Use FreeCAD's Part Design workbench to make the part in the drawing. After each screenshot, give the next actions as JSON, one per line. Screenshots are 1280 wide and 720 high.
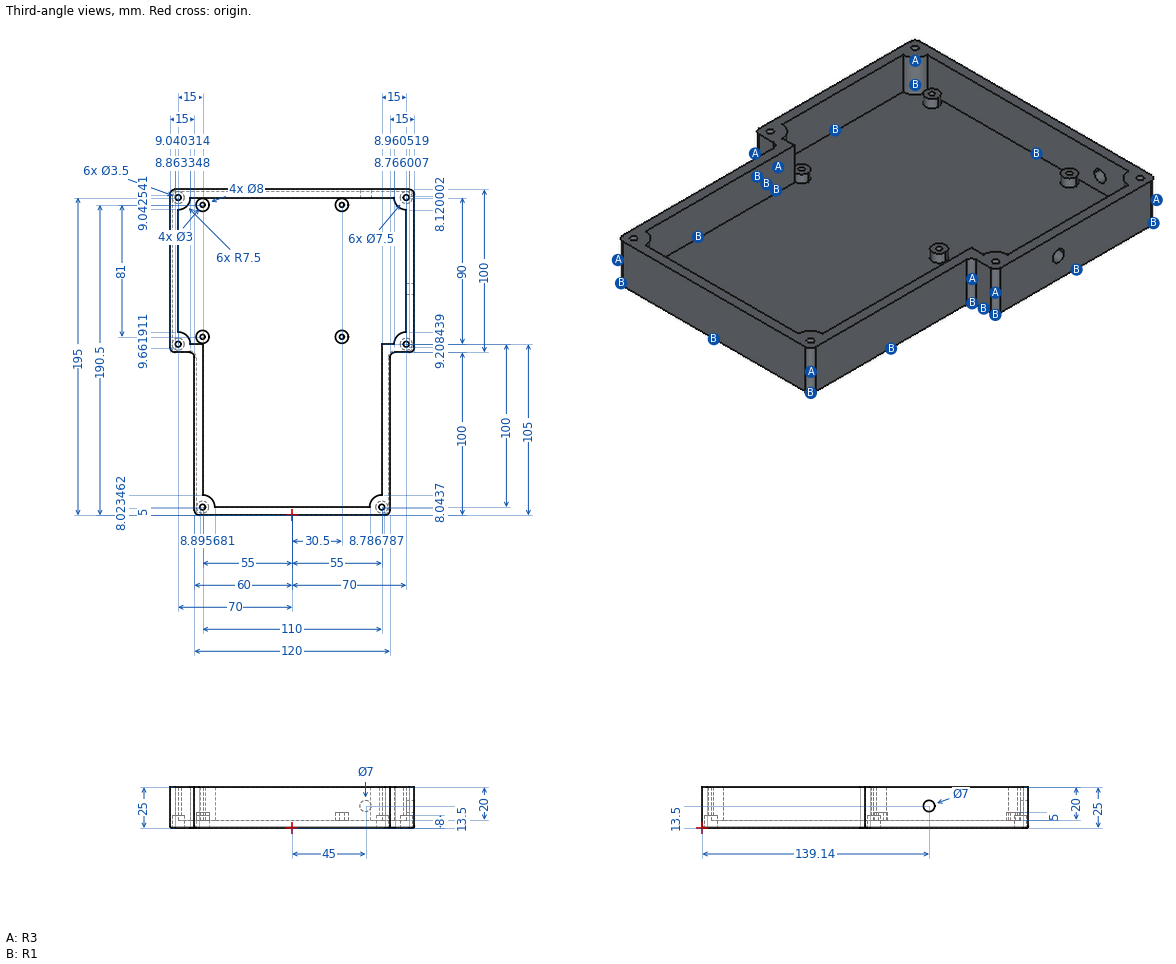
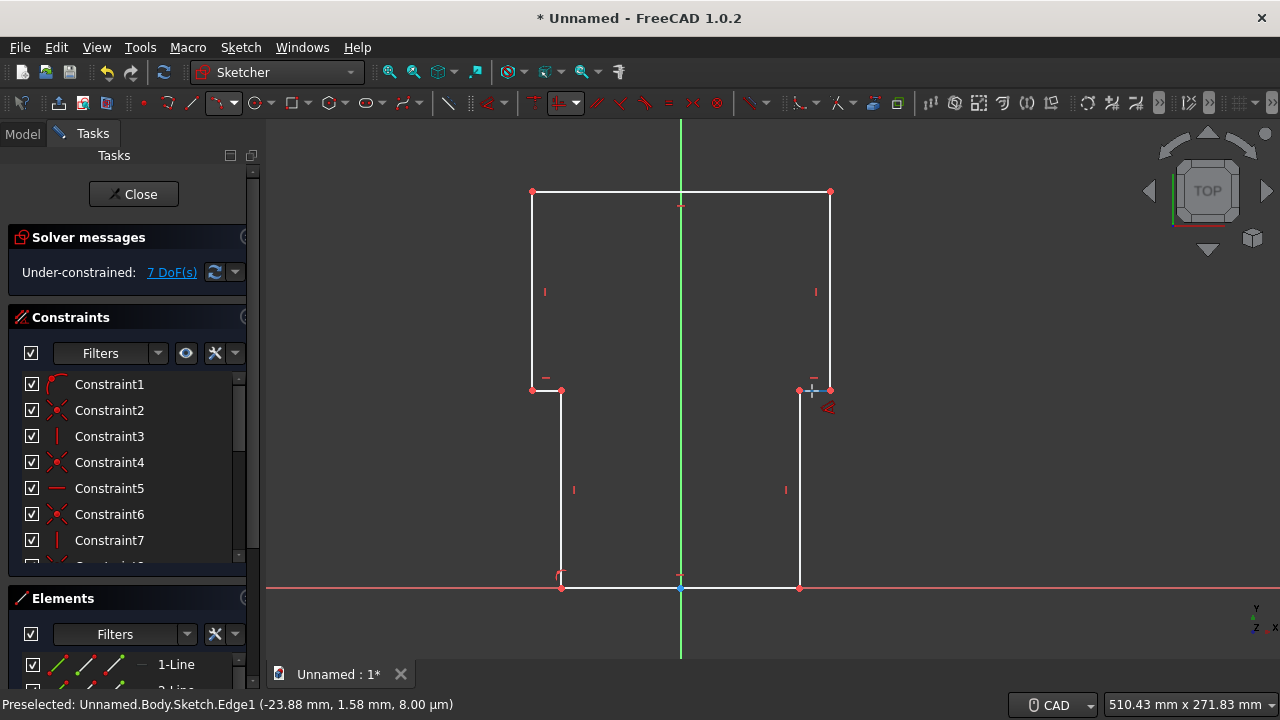
{"action": "left_click", "coordinate": [812, 391]}
{"action": "left_click", "coordinate": [816, 425]}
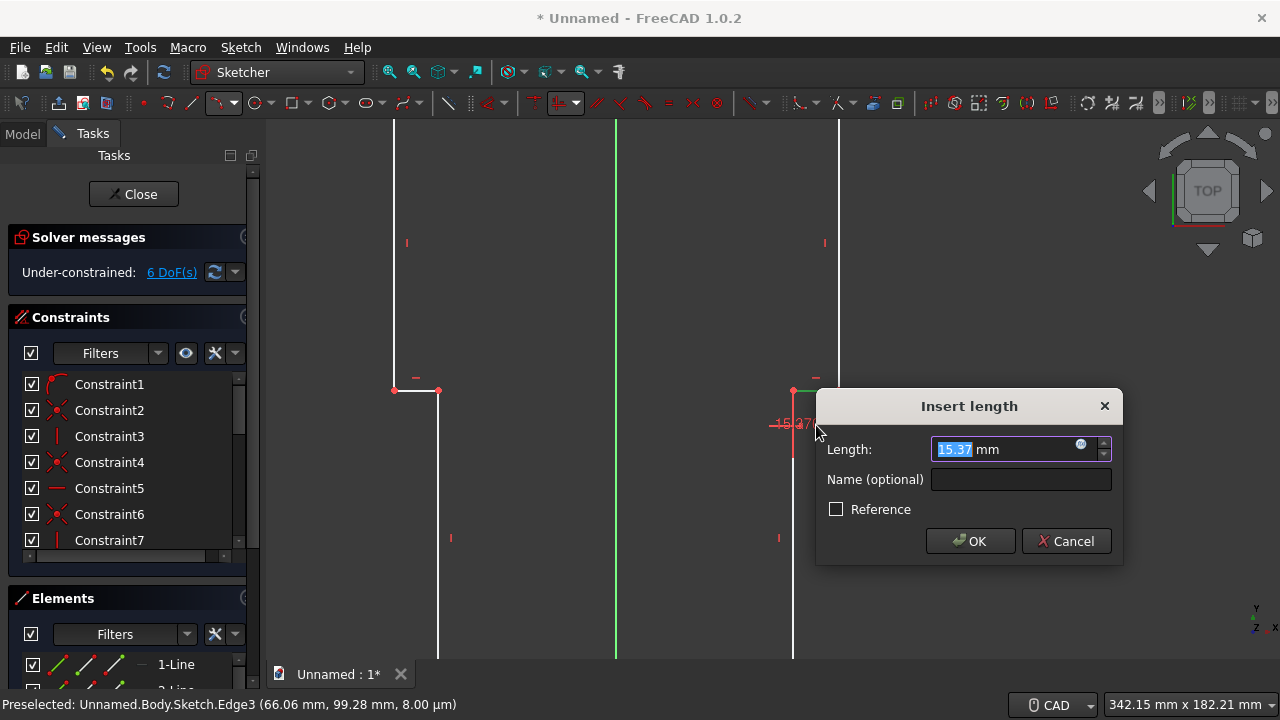
{"action": "type", "text": "15"}
{"action": "key", "text": "Return"}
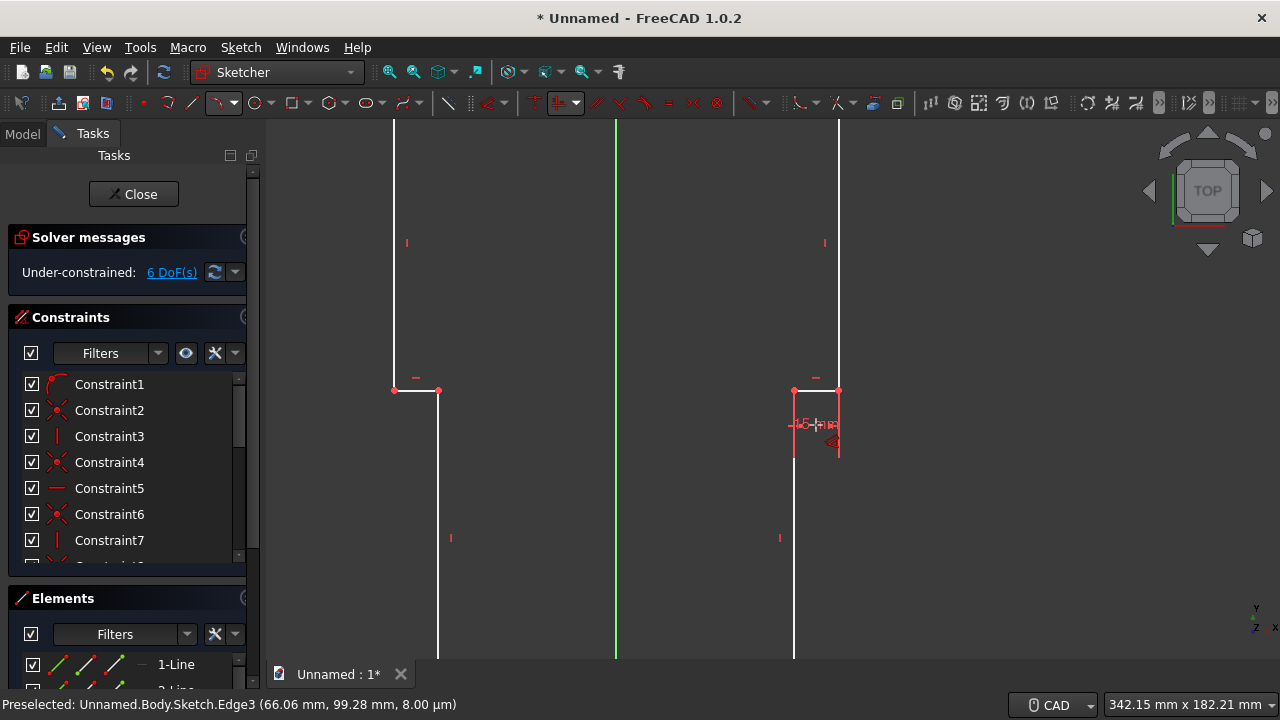
{"action": "left_click", "coordinate": [407, 391]}
{"action": "left_click", "coordinate": [416, 425]}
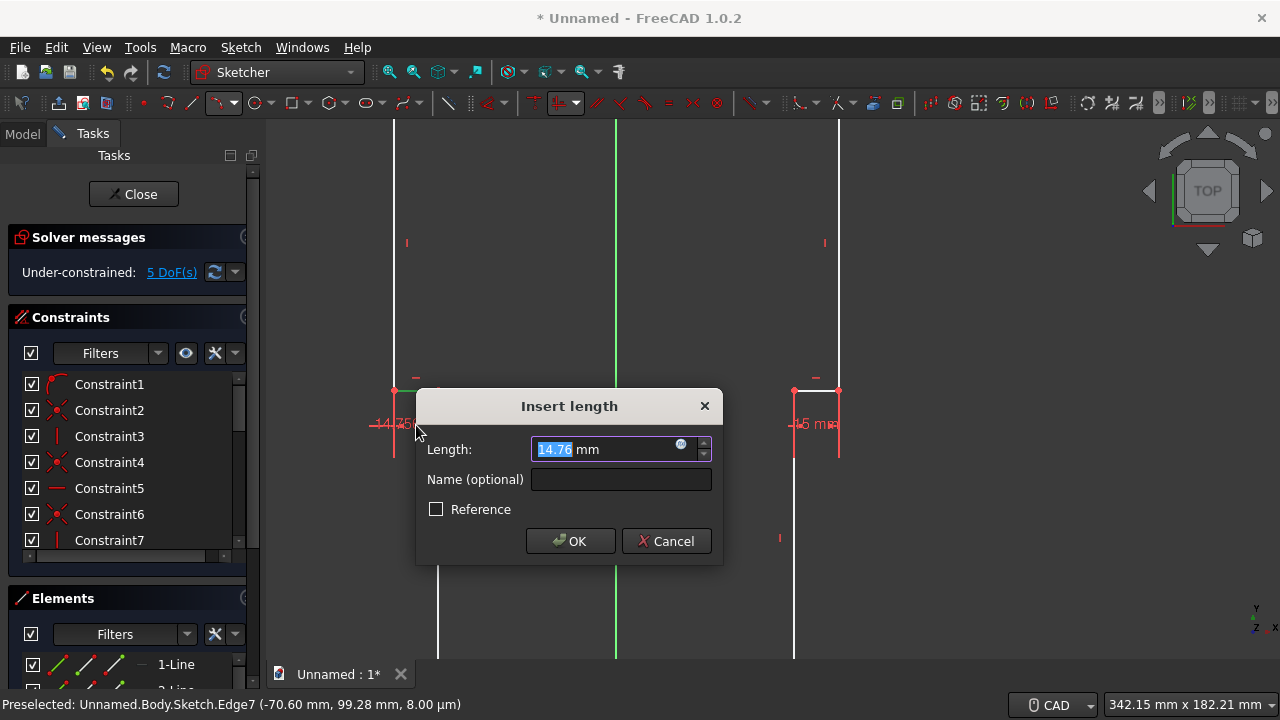
{"action": "type", "text": "15"}
{"action": "key", "text": "Return"}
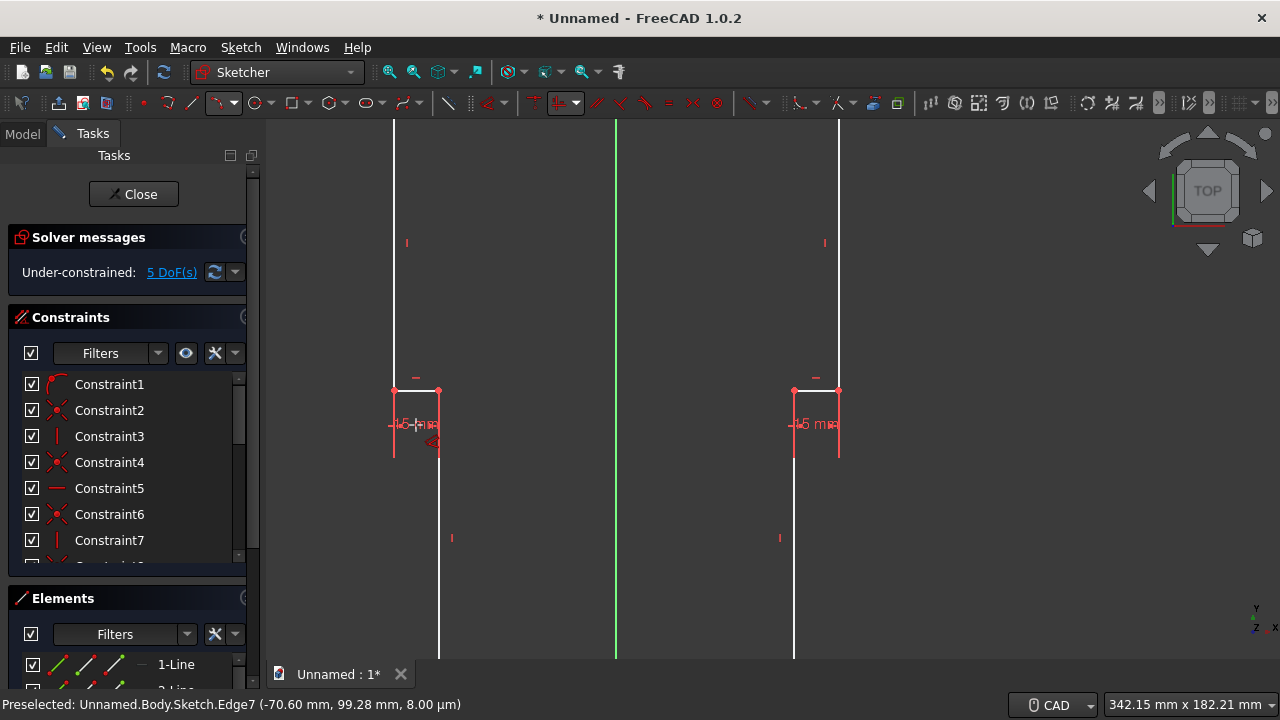
{"action": "scroll", "coordinate": [812, 390], "scroll_direction": "down", "scroll_amount": 3}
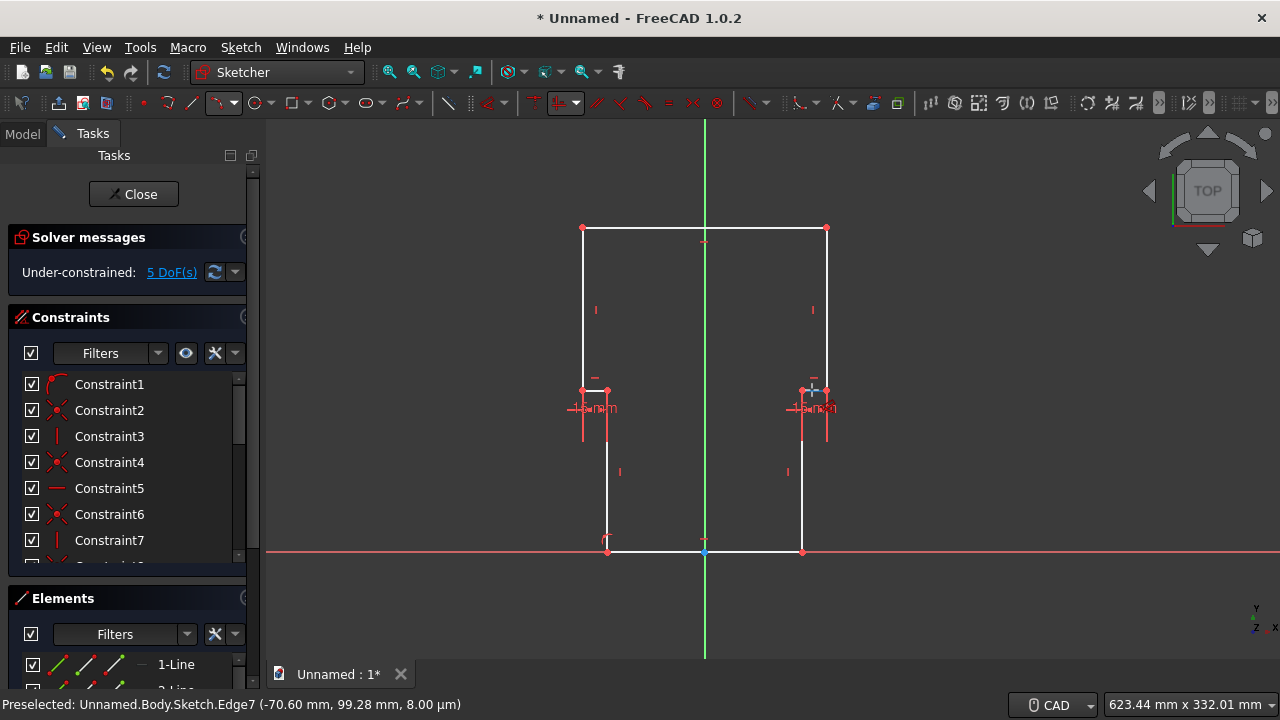
{"action": "left_click", "coordinate": [666, 552]}
{"action": "left_click", "coordinate": [660, 586]}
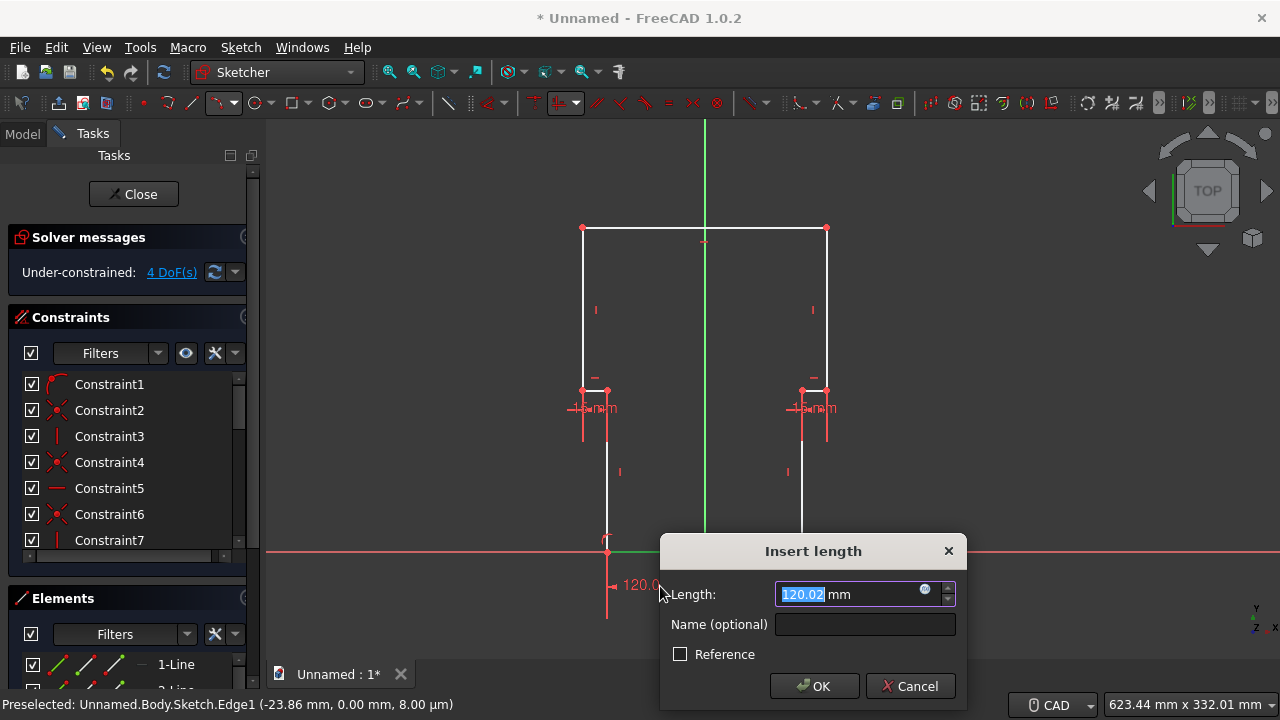
{"action": "type", "text": "120"}
{"action": "key", "text": "Return"}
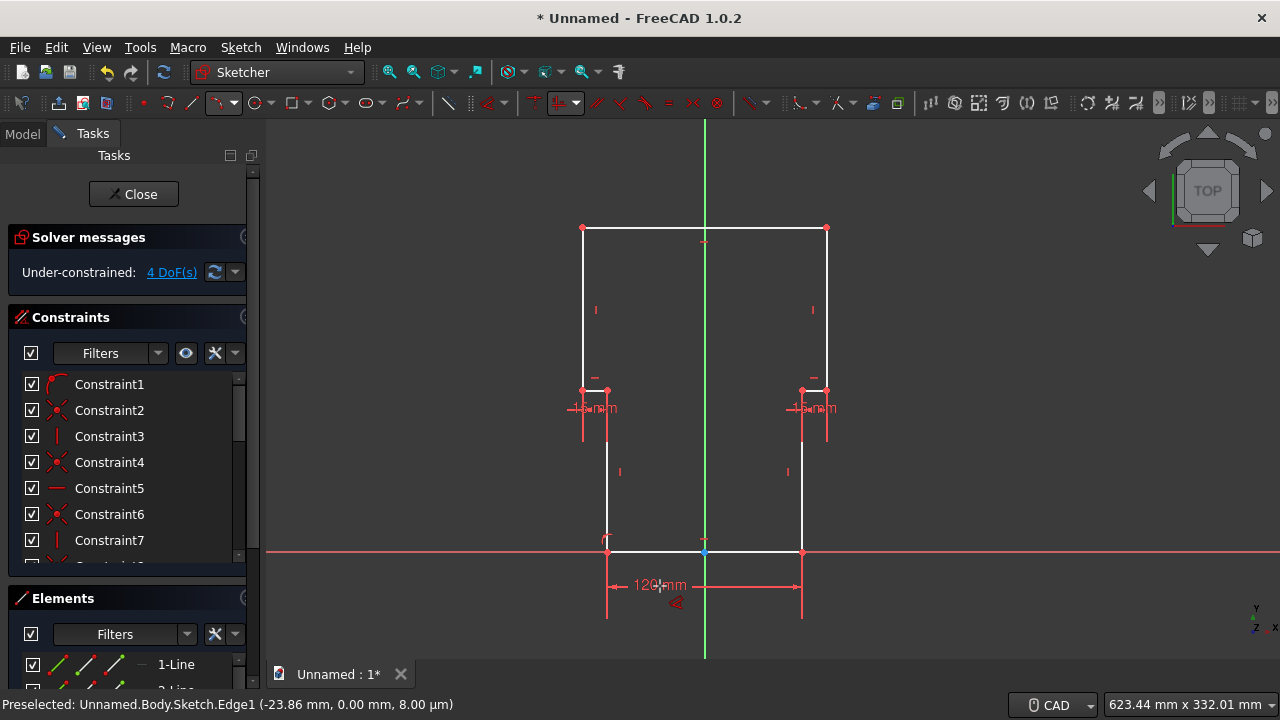
{"action": "left_click", "coordinate": [802, 504]}
{"action": "left_click", "coordinate": [836, 471]}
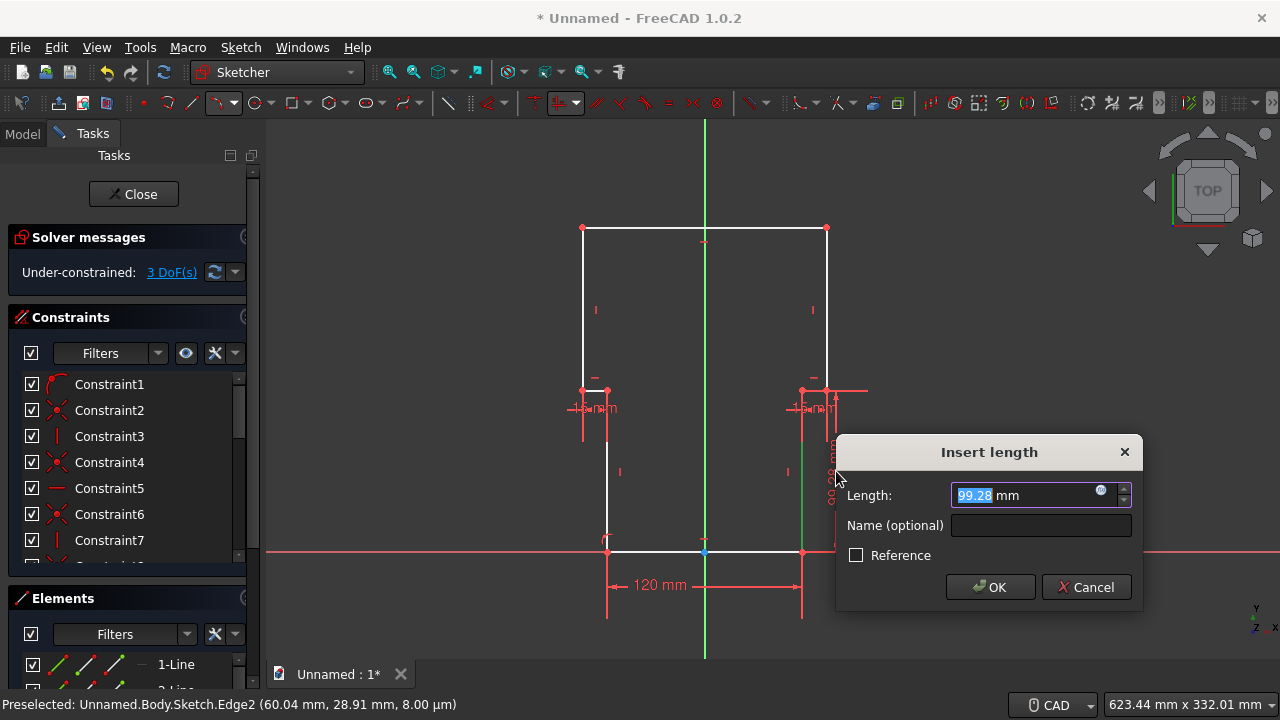
{"action": "type", "text": "100"}
{"action": "key", "text": "Return"}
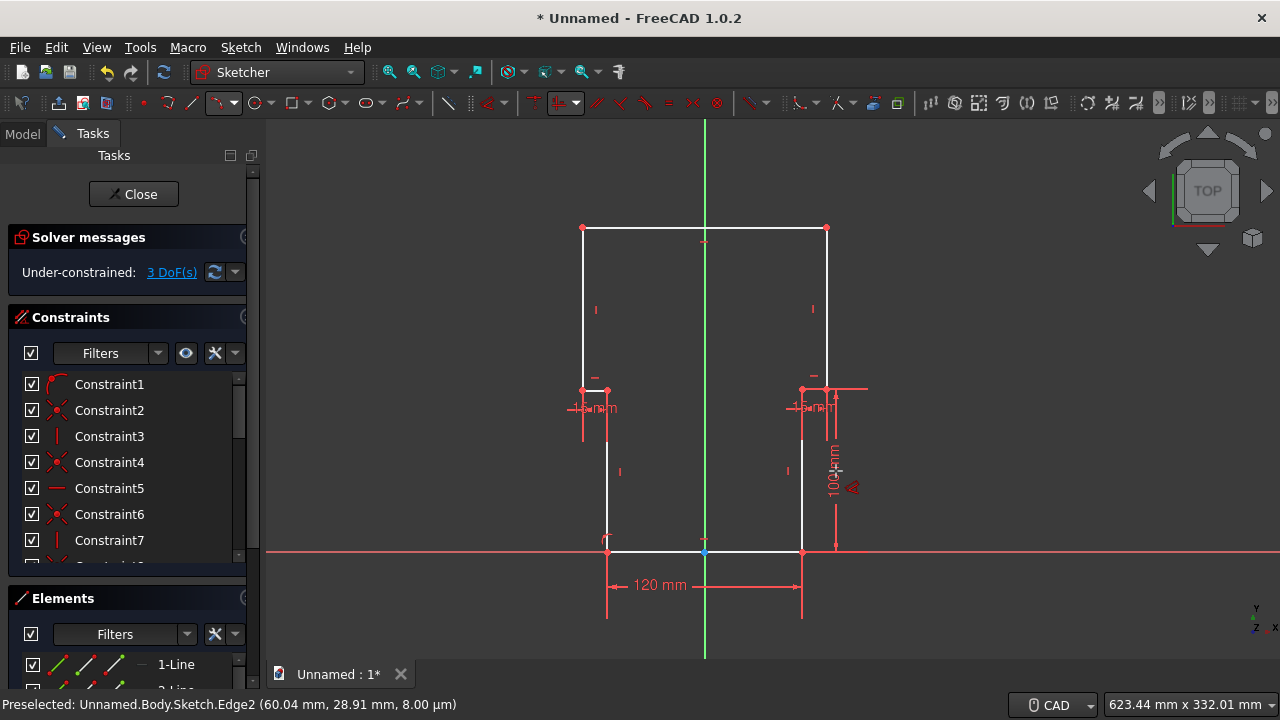
{"action": "left_click", "coordinate": [827, 341]}
{"action": "left_click", "coordinate": [861, 308]}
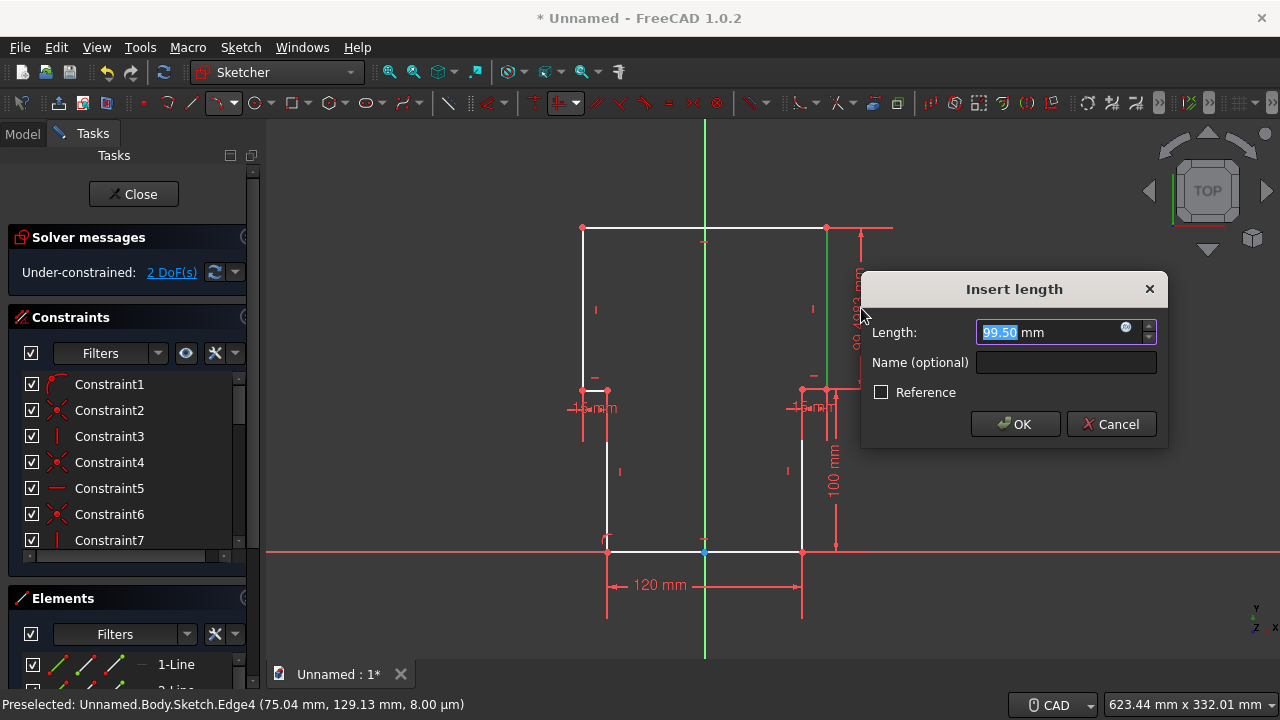
{"action": "type", "text": "100"}
{"action": "key", "text": "Return"}